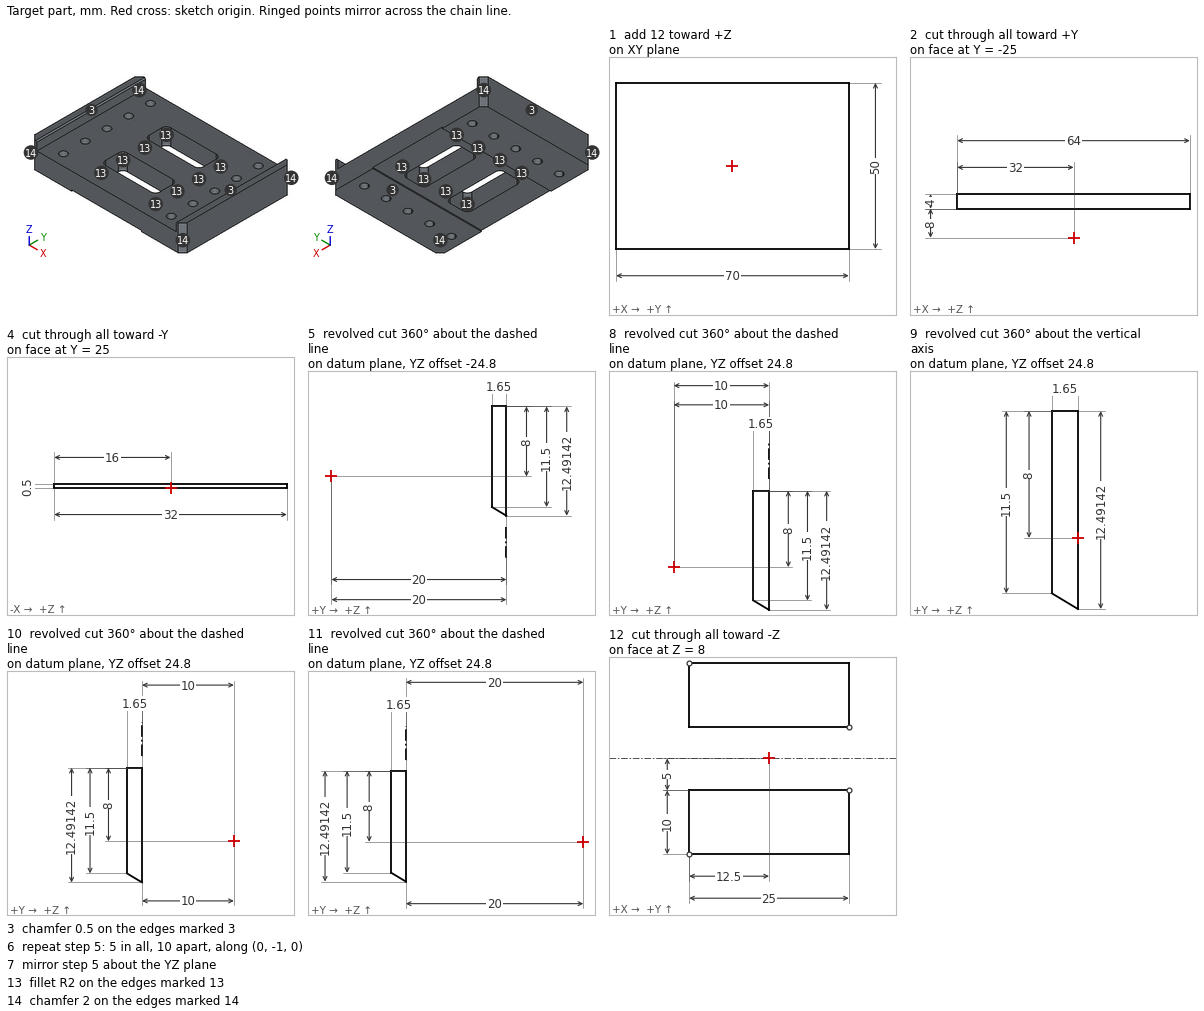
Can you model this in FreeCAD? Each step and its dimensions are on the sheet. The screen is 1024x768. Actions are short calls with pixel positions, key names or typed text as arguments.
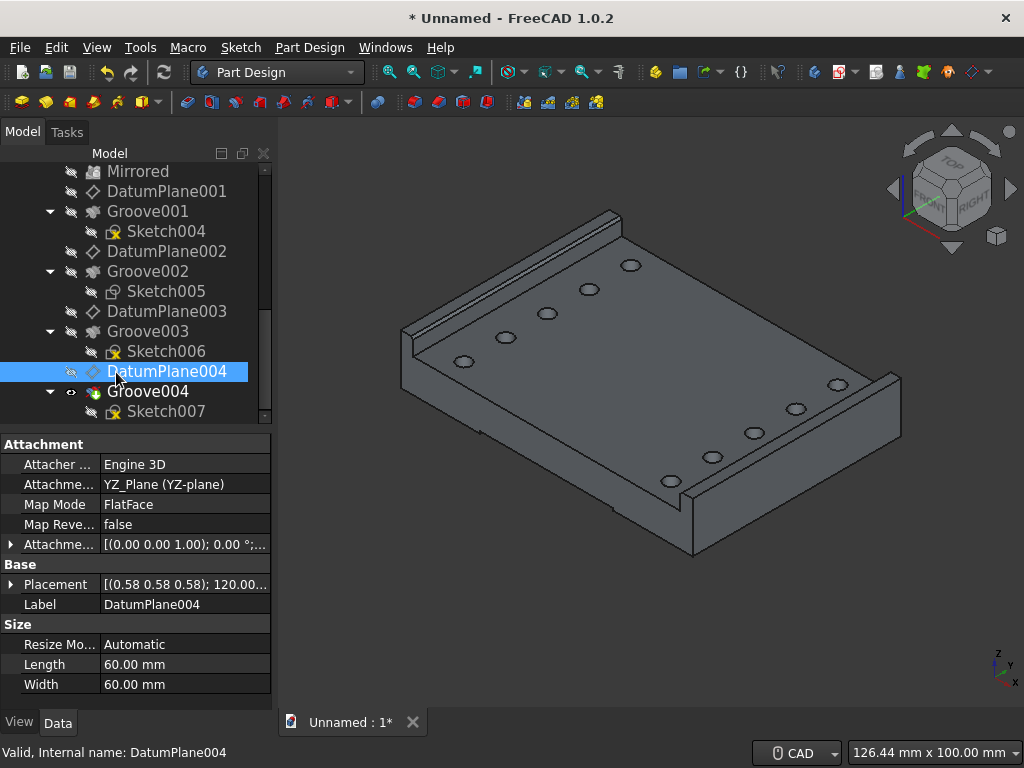
click(651, 372)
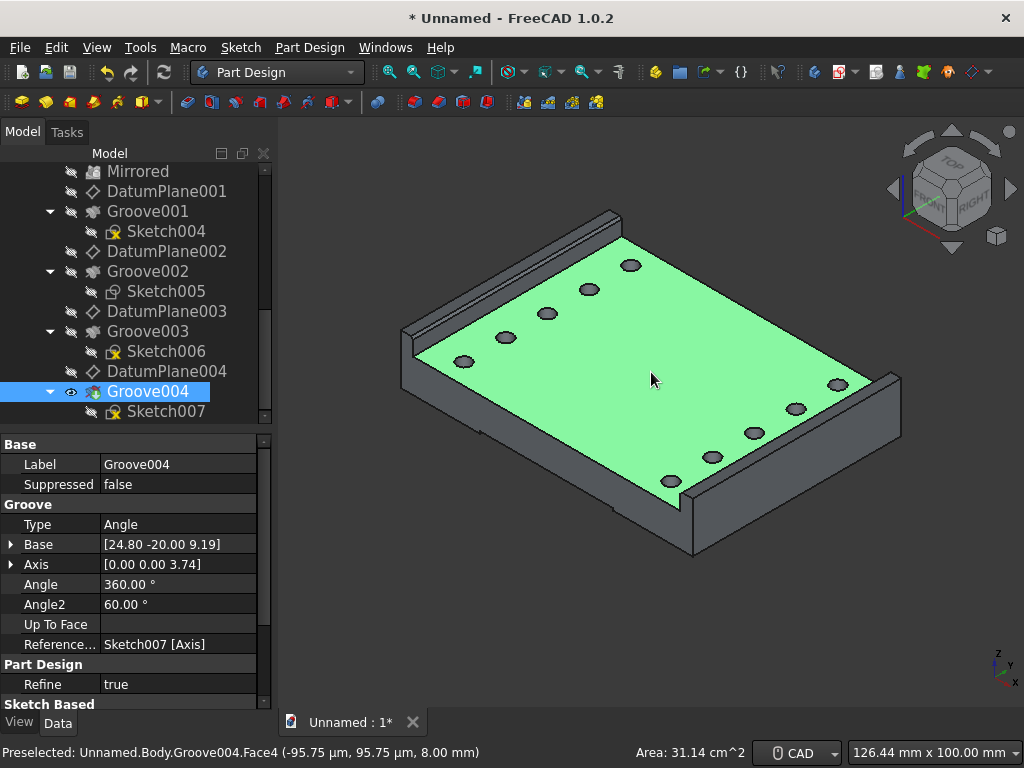
click(840, 72)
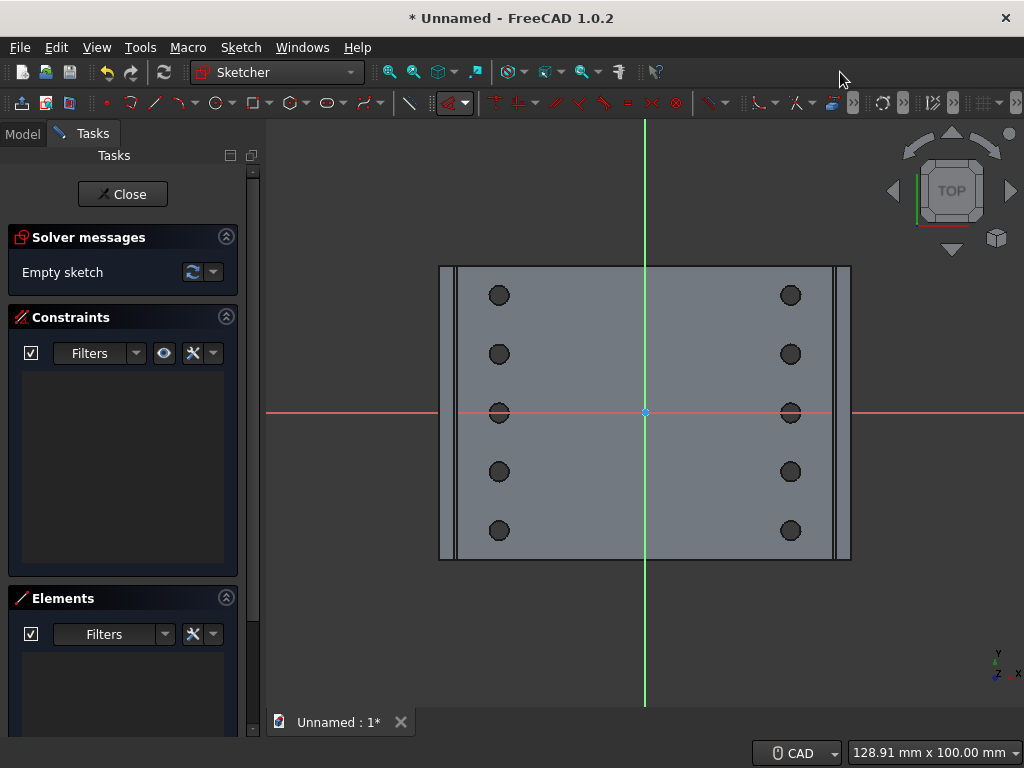
scroll(701, 413, up, 4)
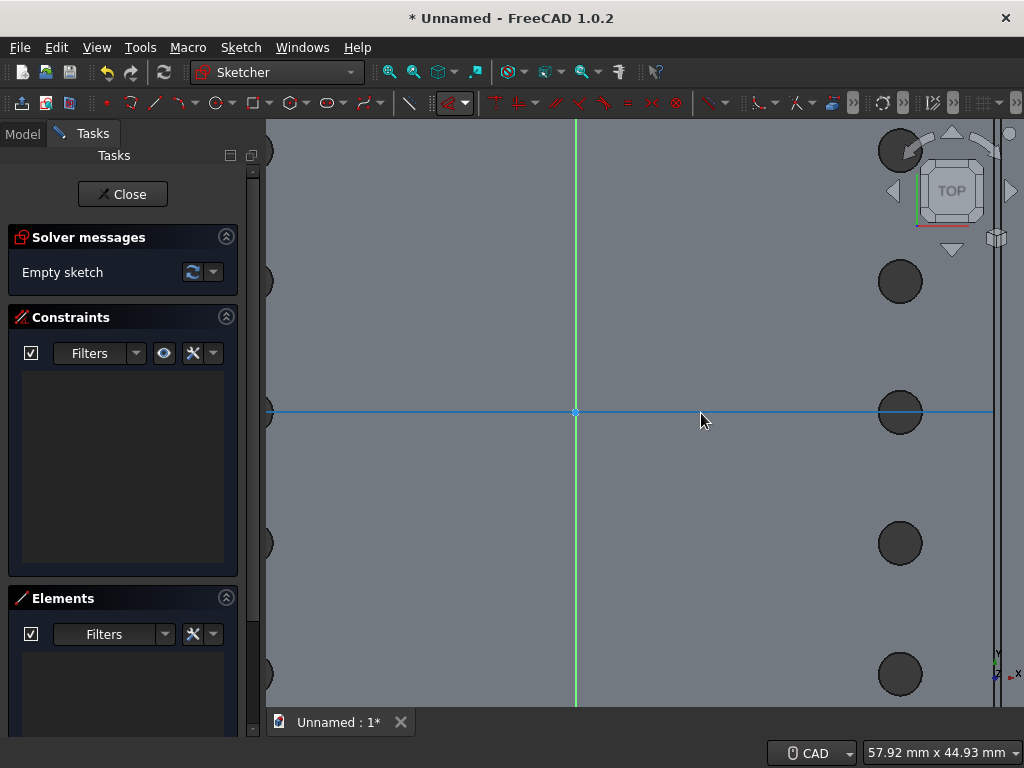
key(g)
key(r)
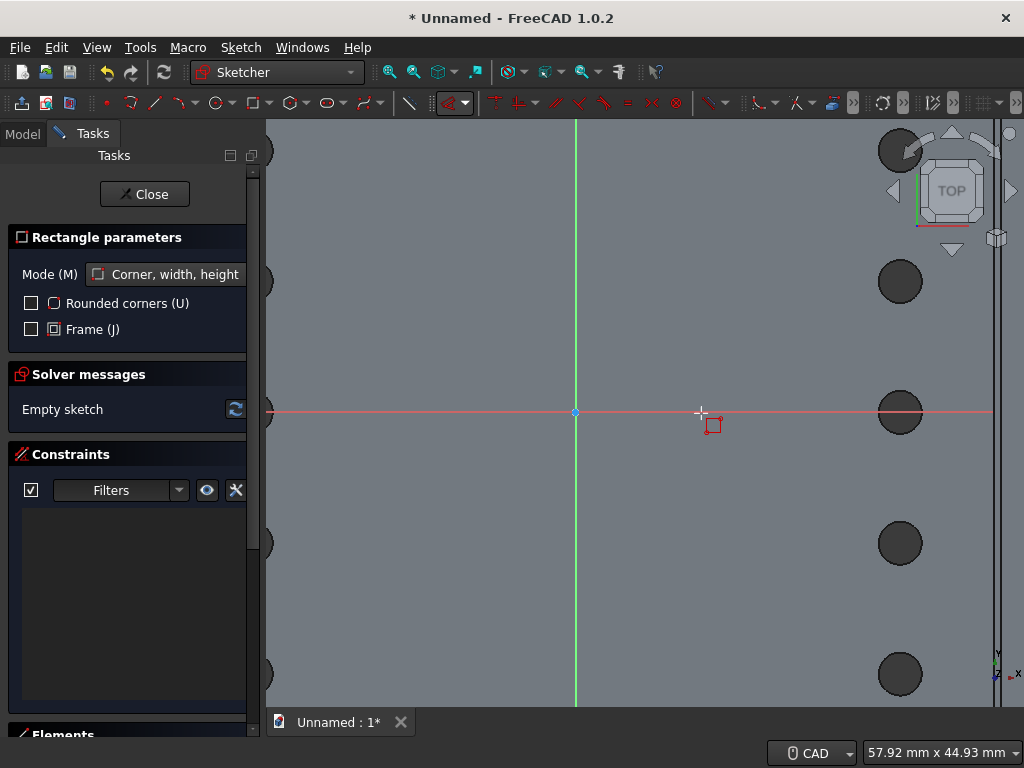
click(412, 478)
click(739, 609)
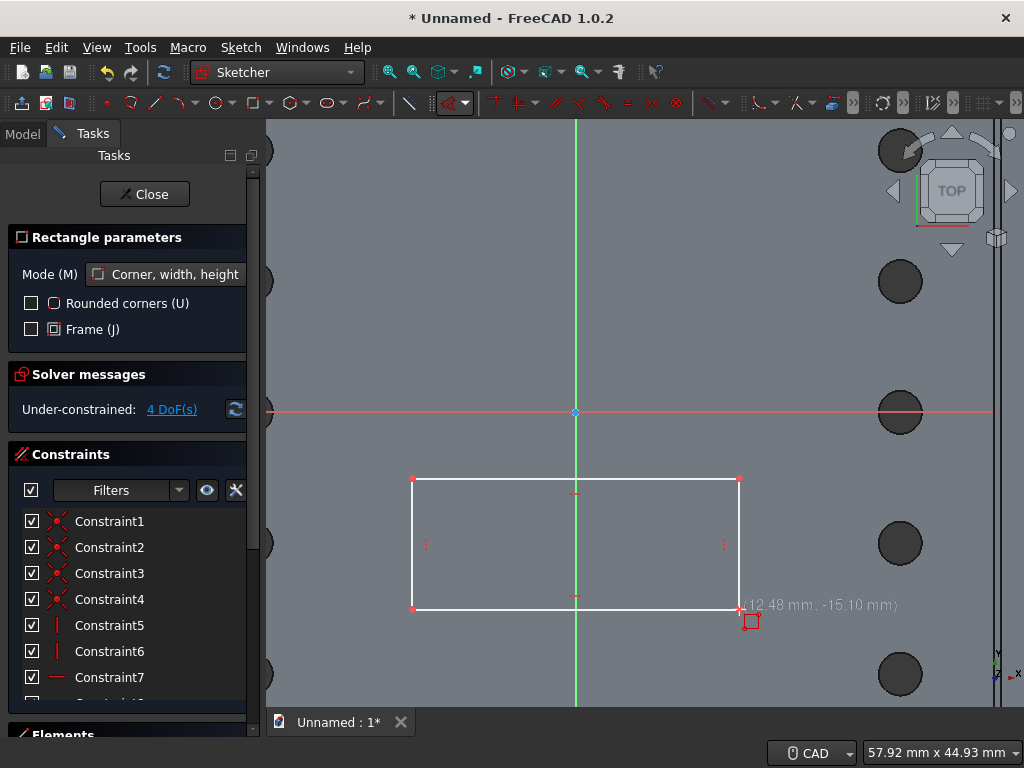
click(412, 216)
click(739, 347)
key(Escape)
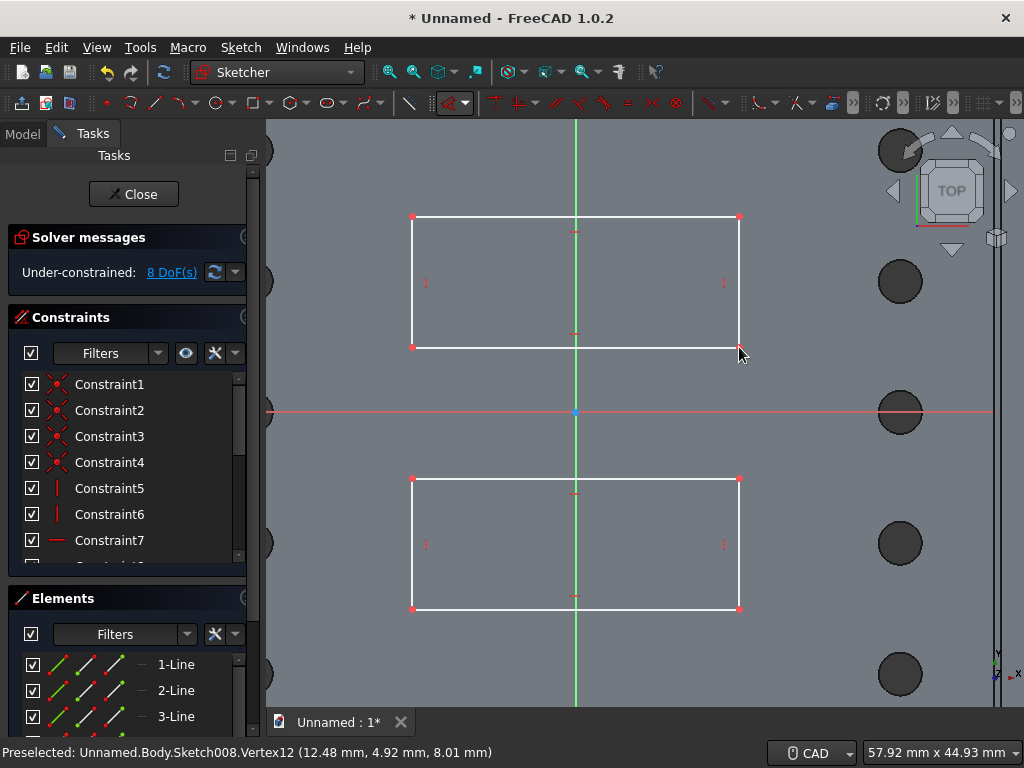
click(412, 610)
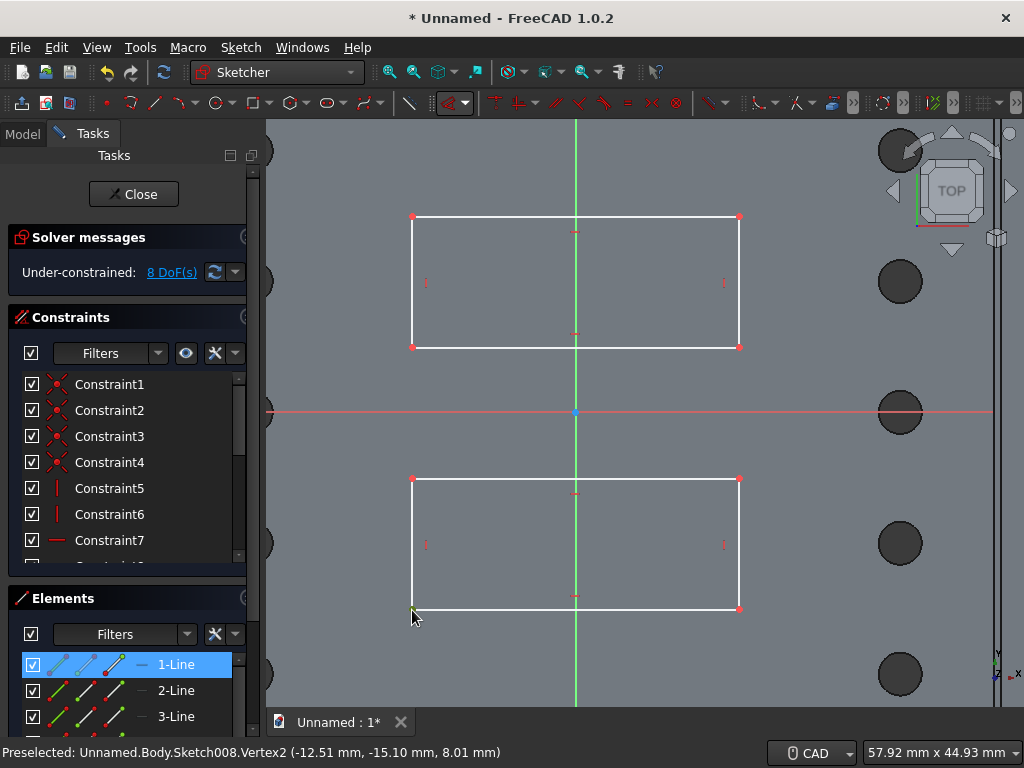
click(412, 217)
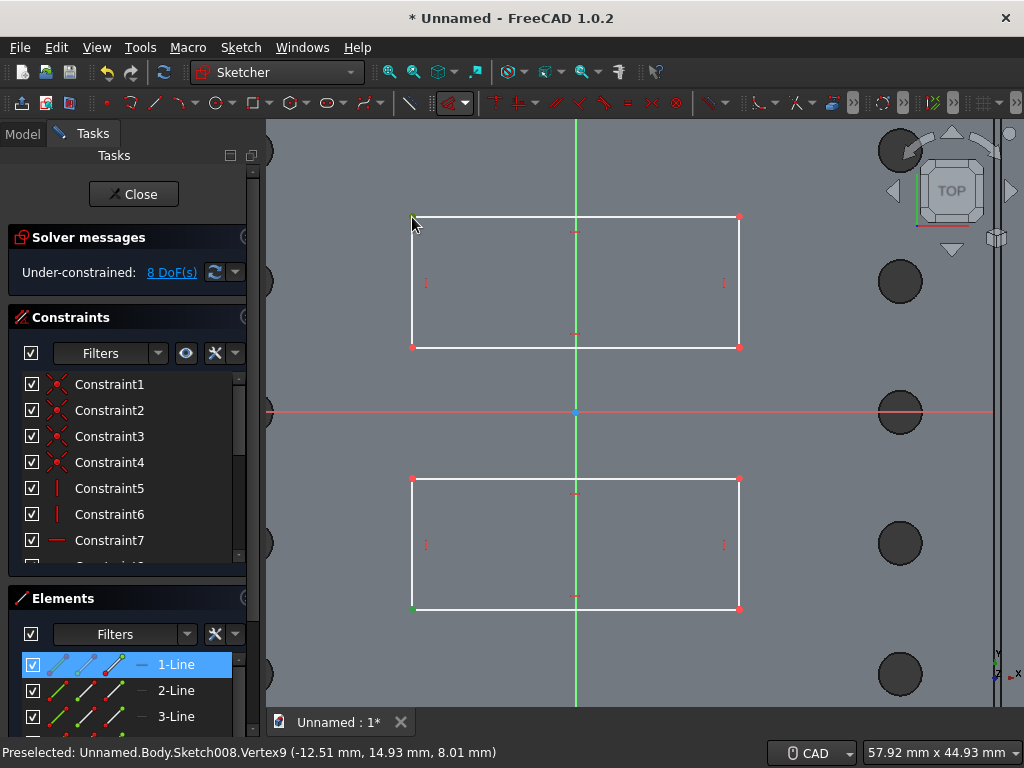
click(334, 412)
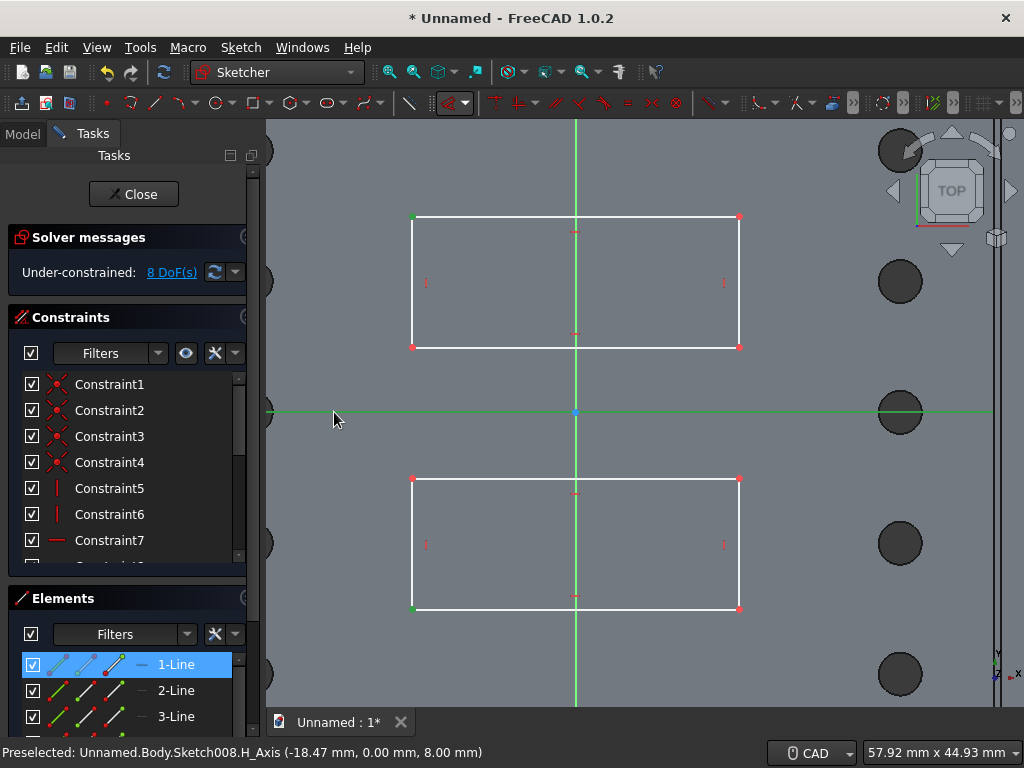
click(652, 104)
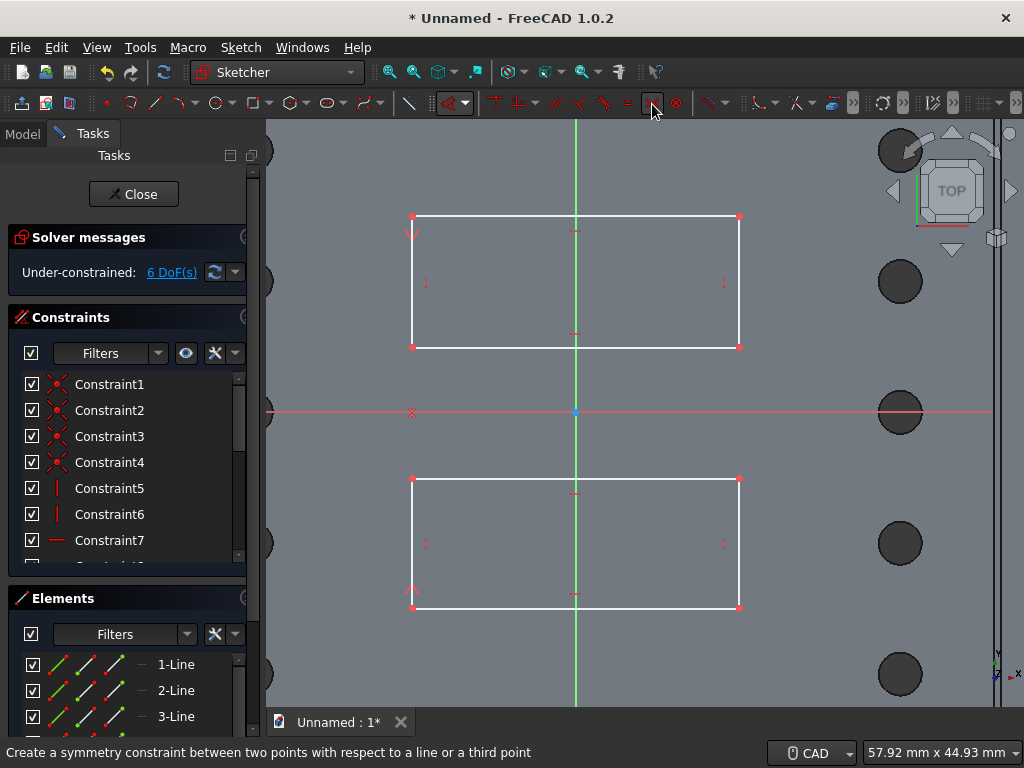
click(739, 479)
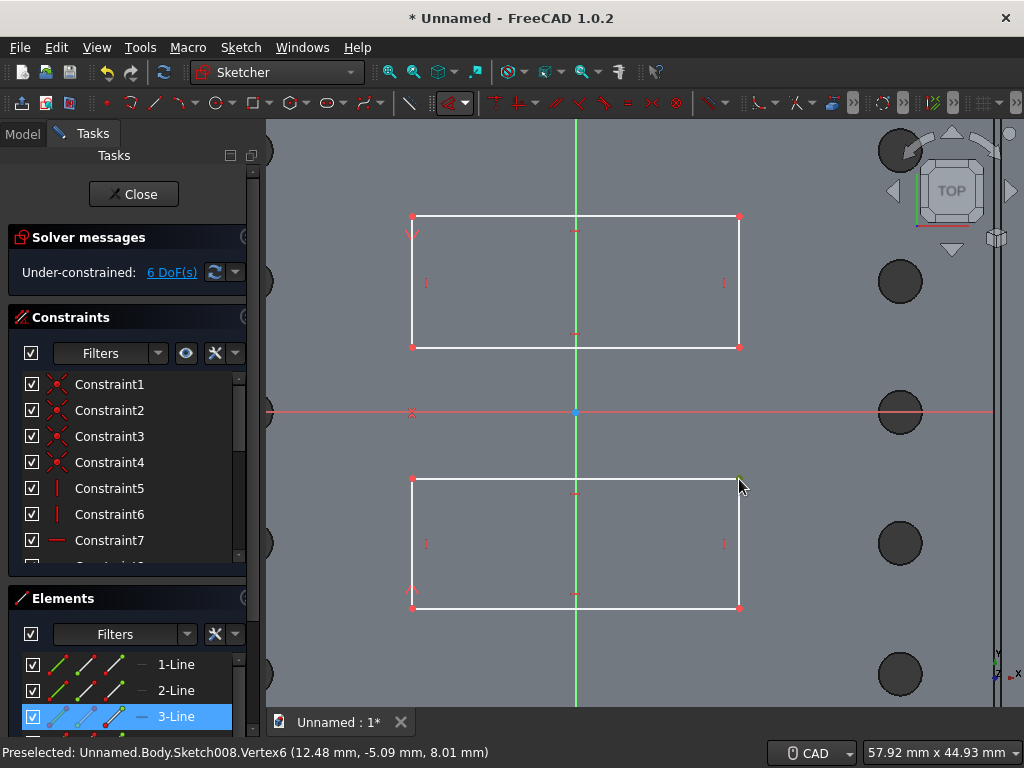
click(739, 348)